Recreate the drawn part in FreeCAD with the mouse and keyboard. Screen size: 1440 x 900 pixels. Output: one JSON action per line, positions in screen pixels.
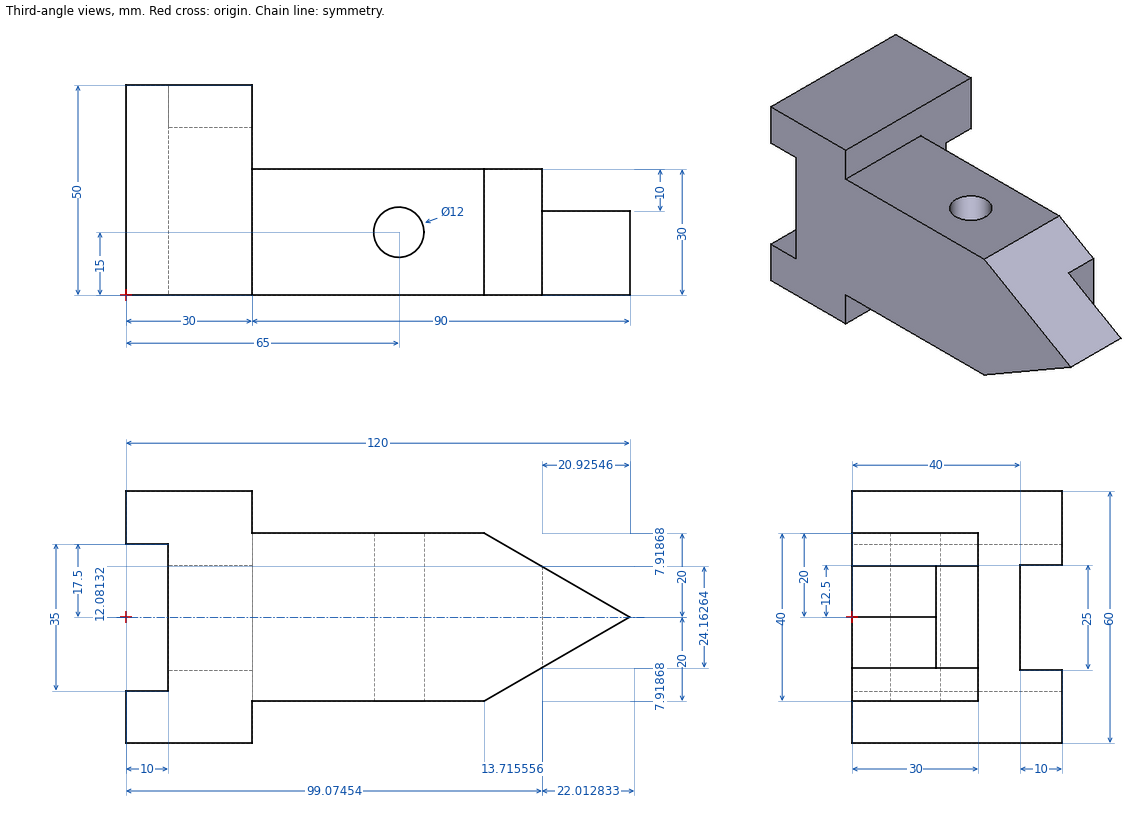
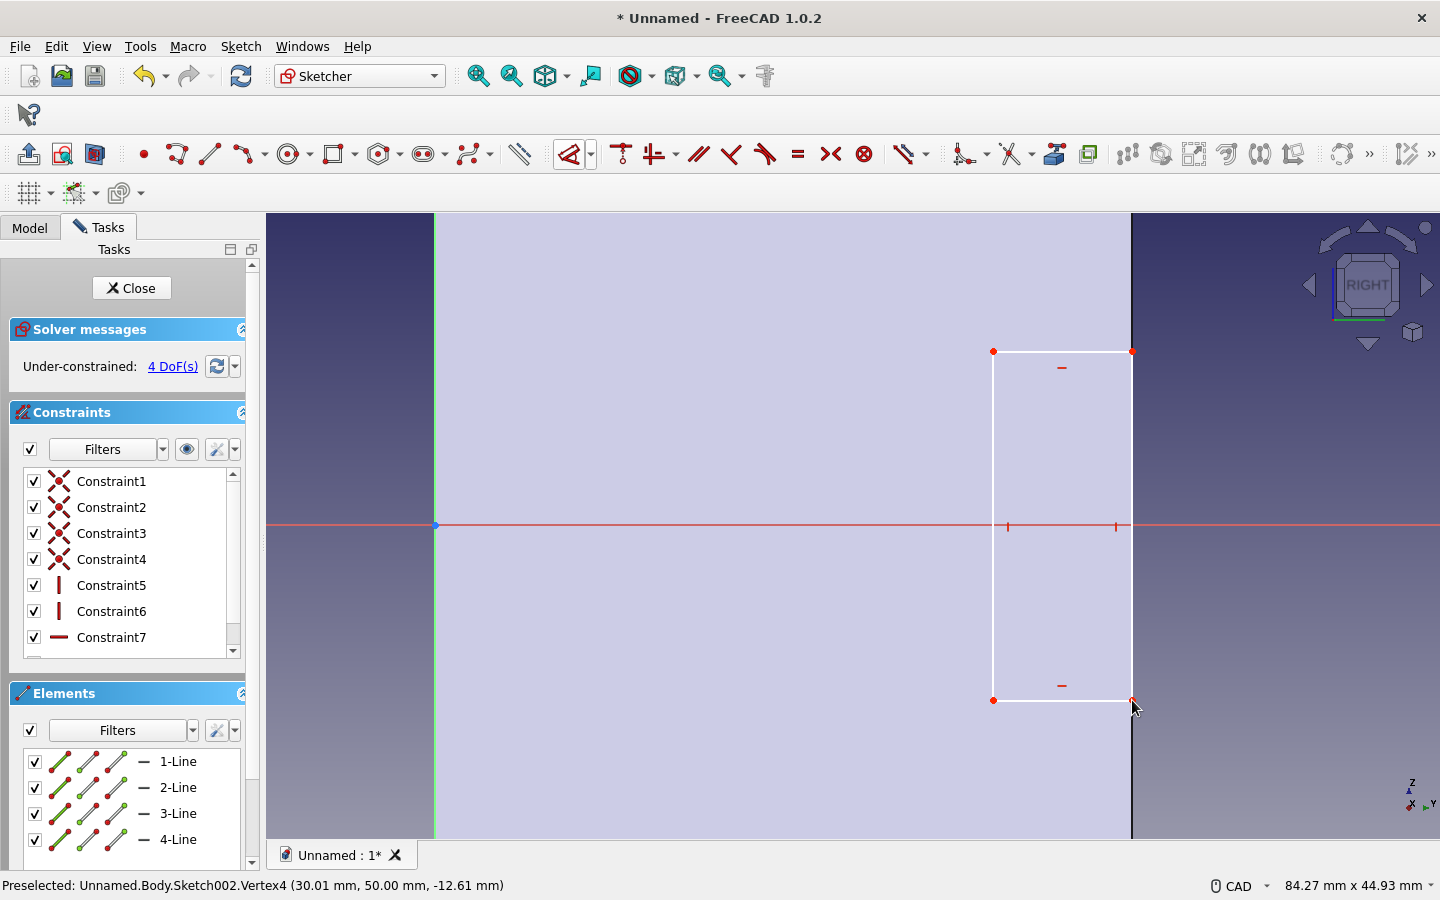
{"action": "left_click", "coordinate": [993, 457]}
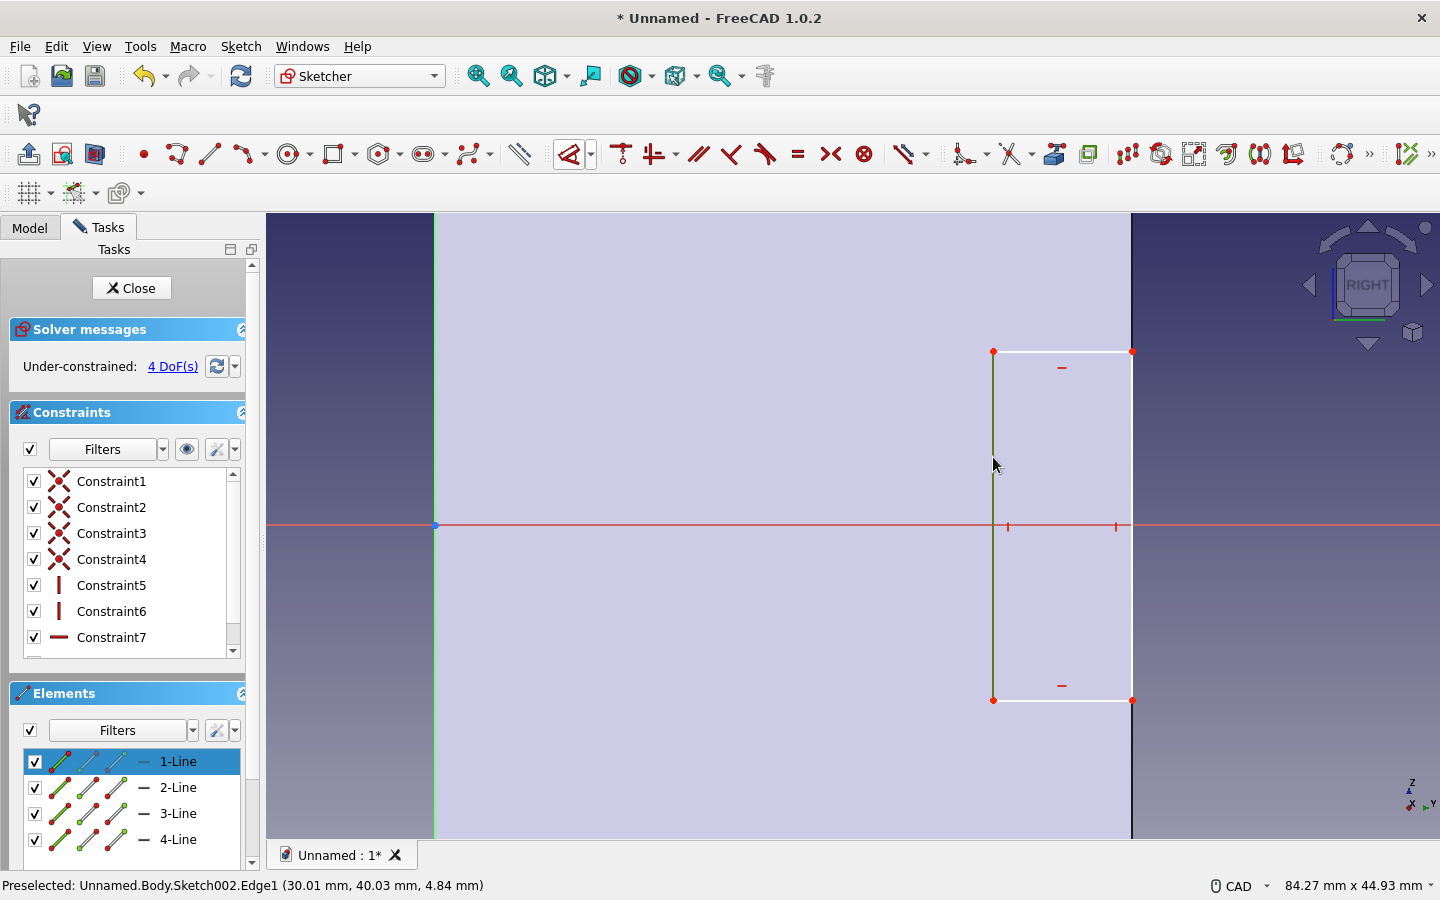
{"action": "left_click", "coordinate": [590, 154]}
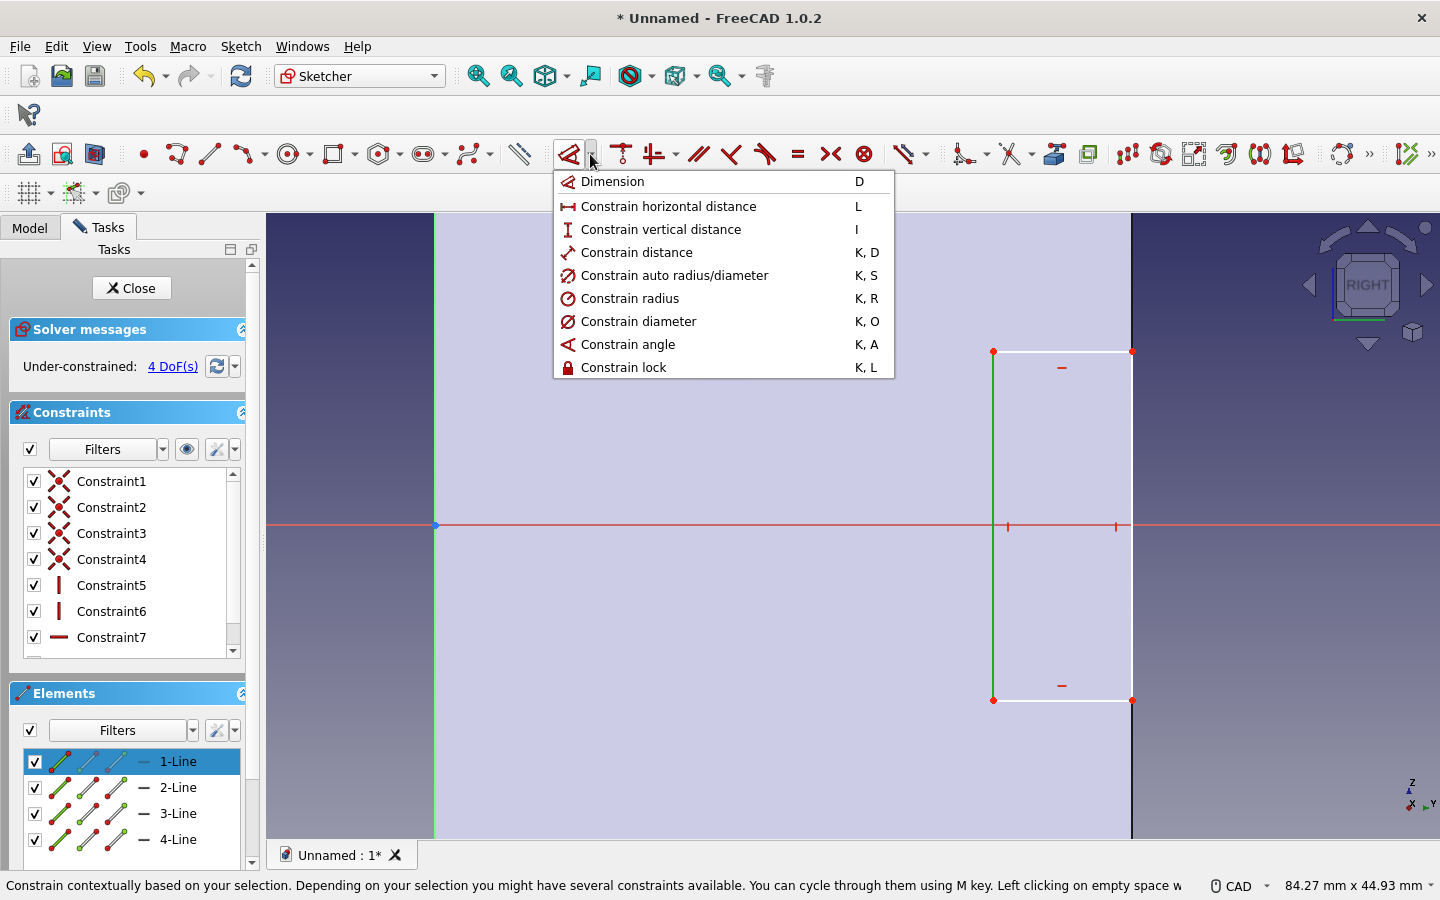
{"action": "left_click", "coordinate": [724, 230]}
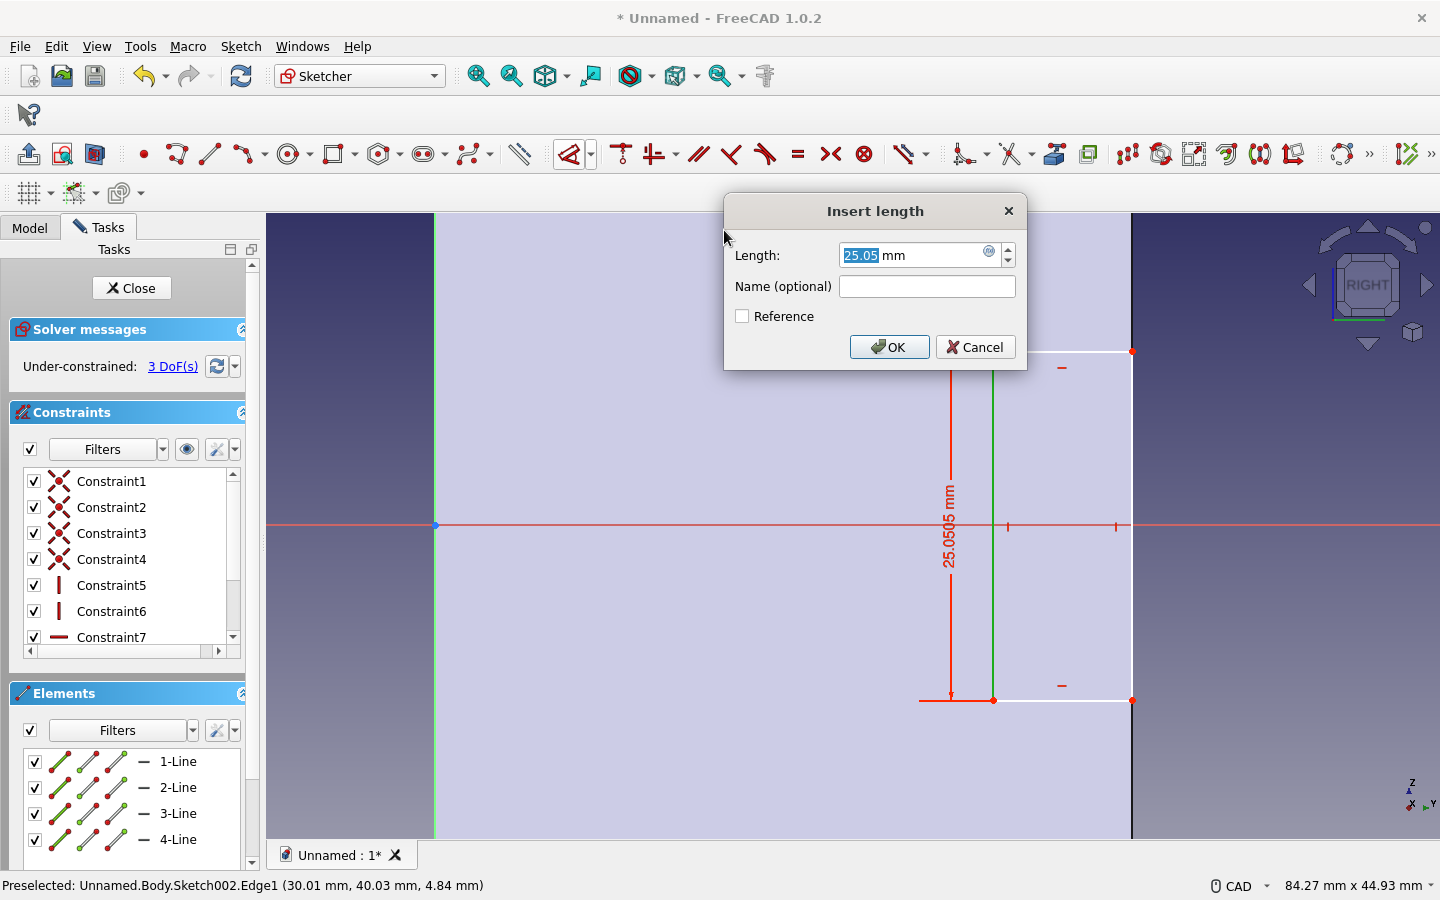
{"action": "type", "text": "25"}
{"action": "key", "text": "Return"}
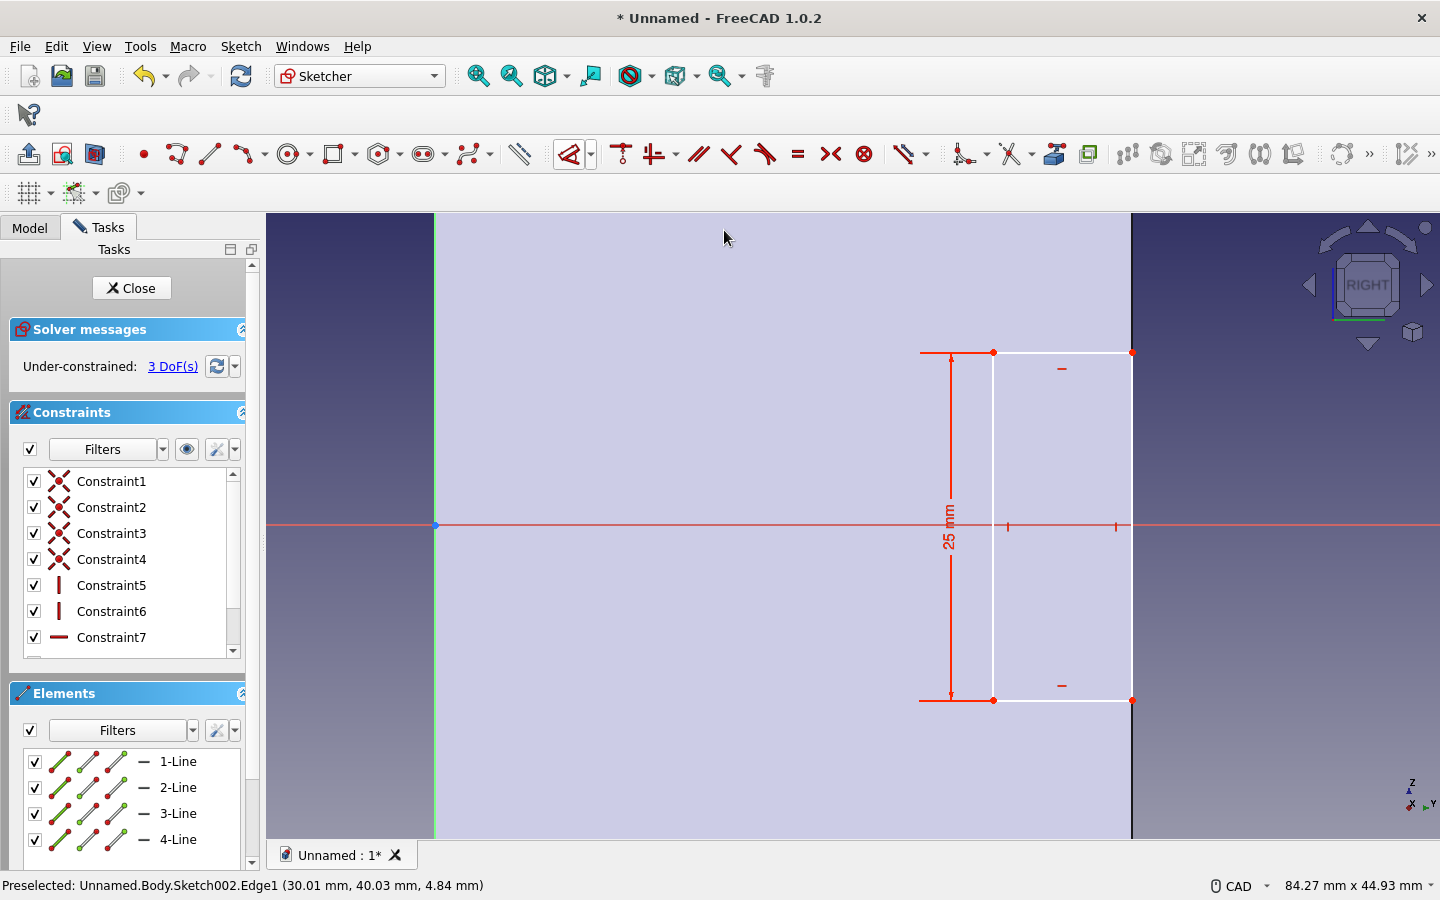
{"action": "left_click", "coordinate": [1035, 701]}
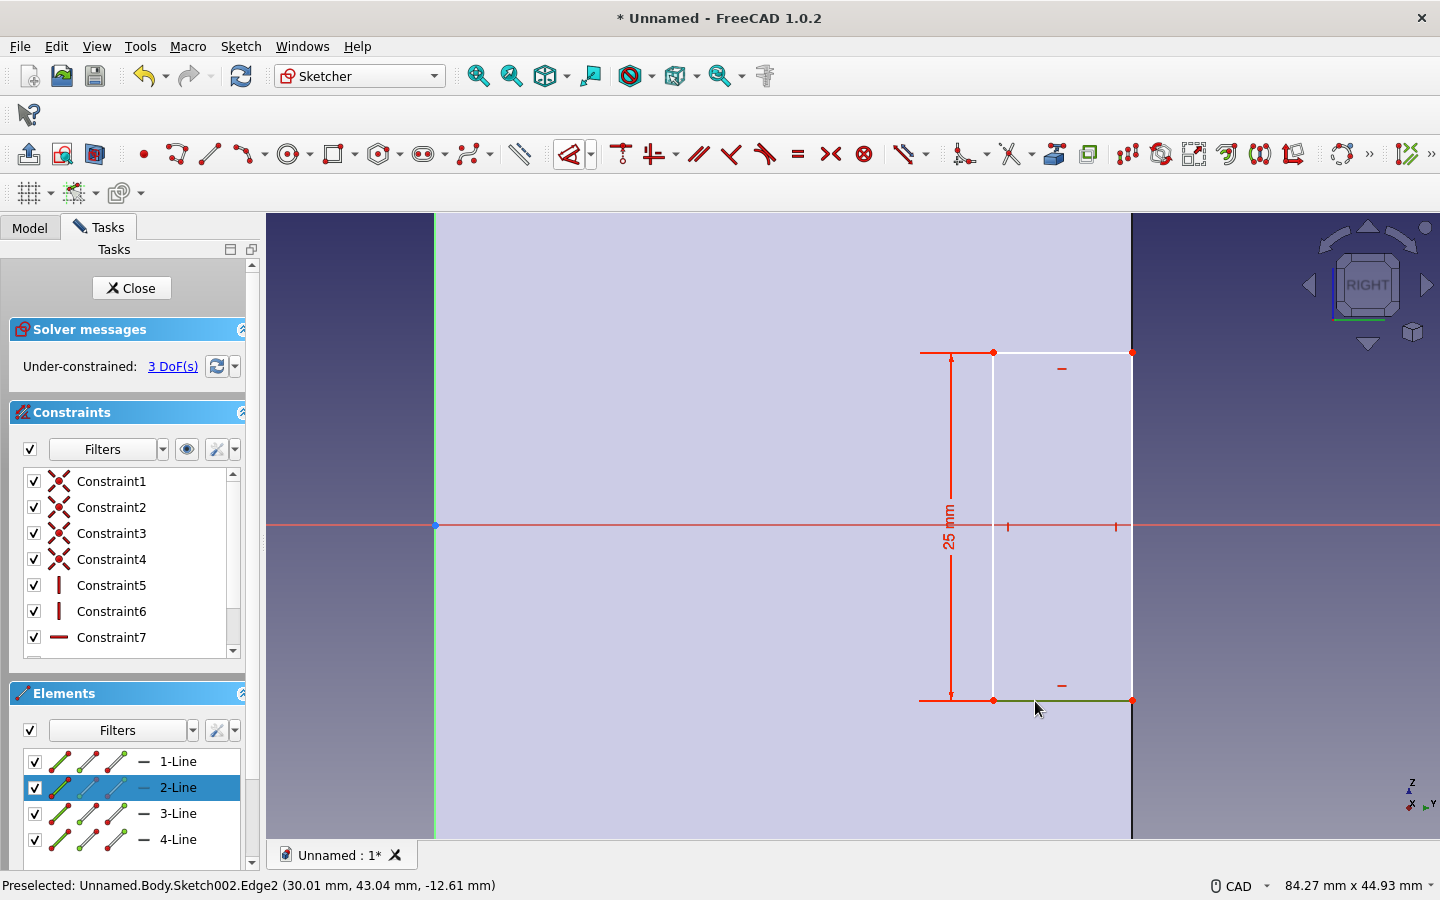
{"action": "left_click", "coordinate": [590, 154]}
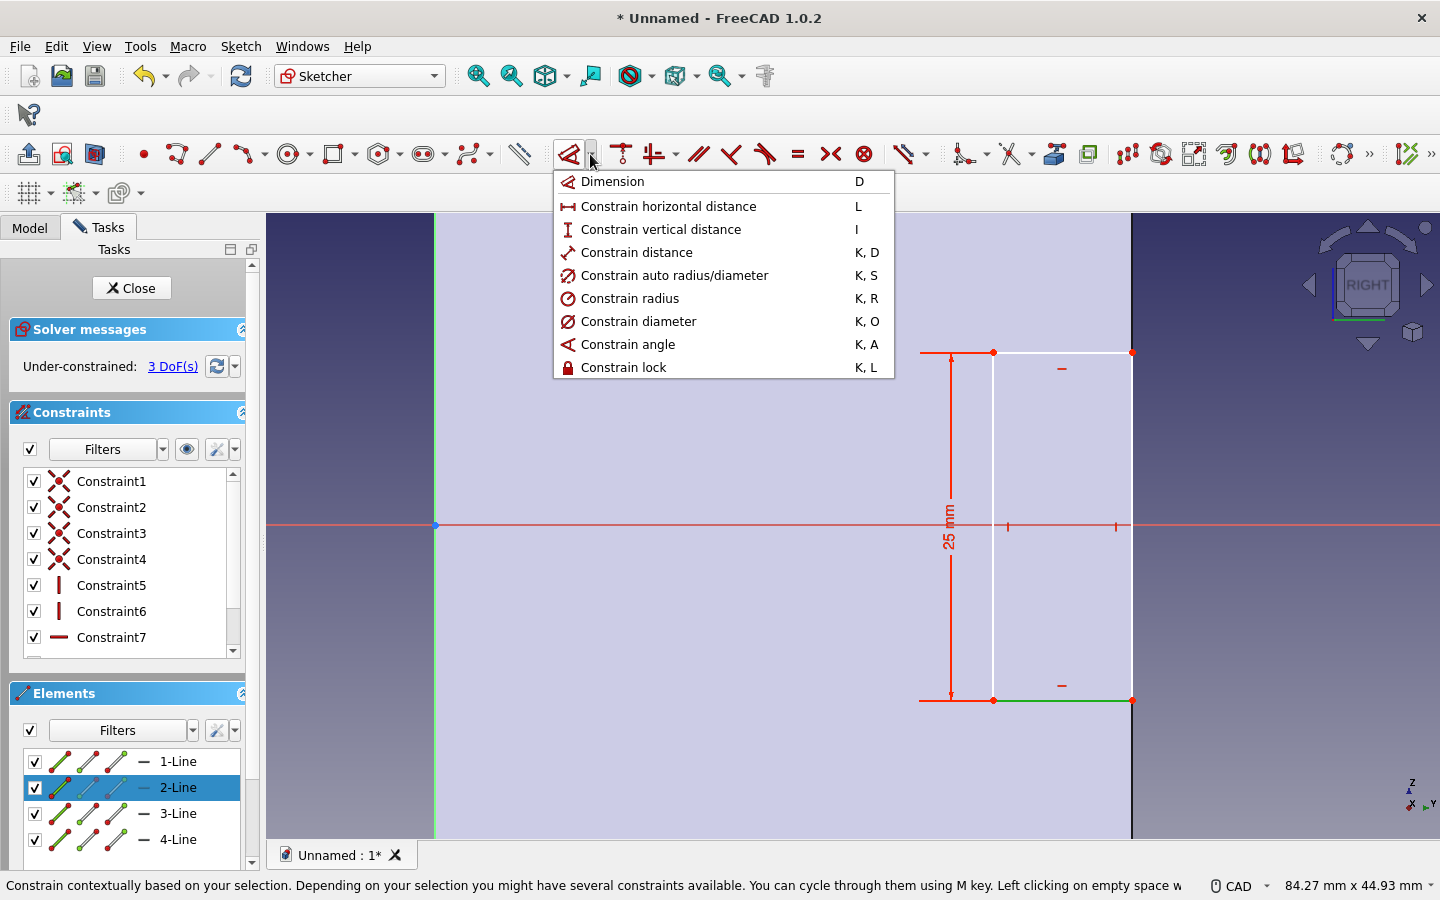
{"action": "left_click", "coordinate": [724, 206]}